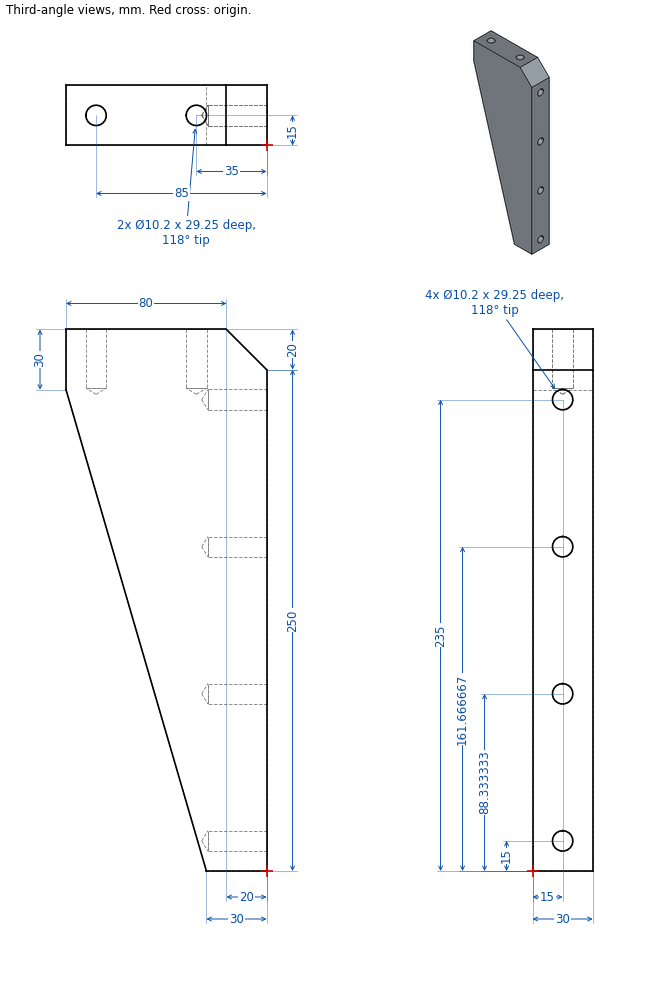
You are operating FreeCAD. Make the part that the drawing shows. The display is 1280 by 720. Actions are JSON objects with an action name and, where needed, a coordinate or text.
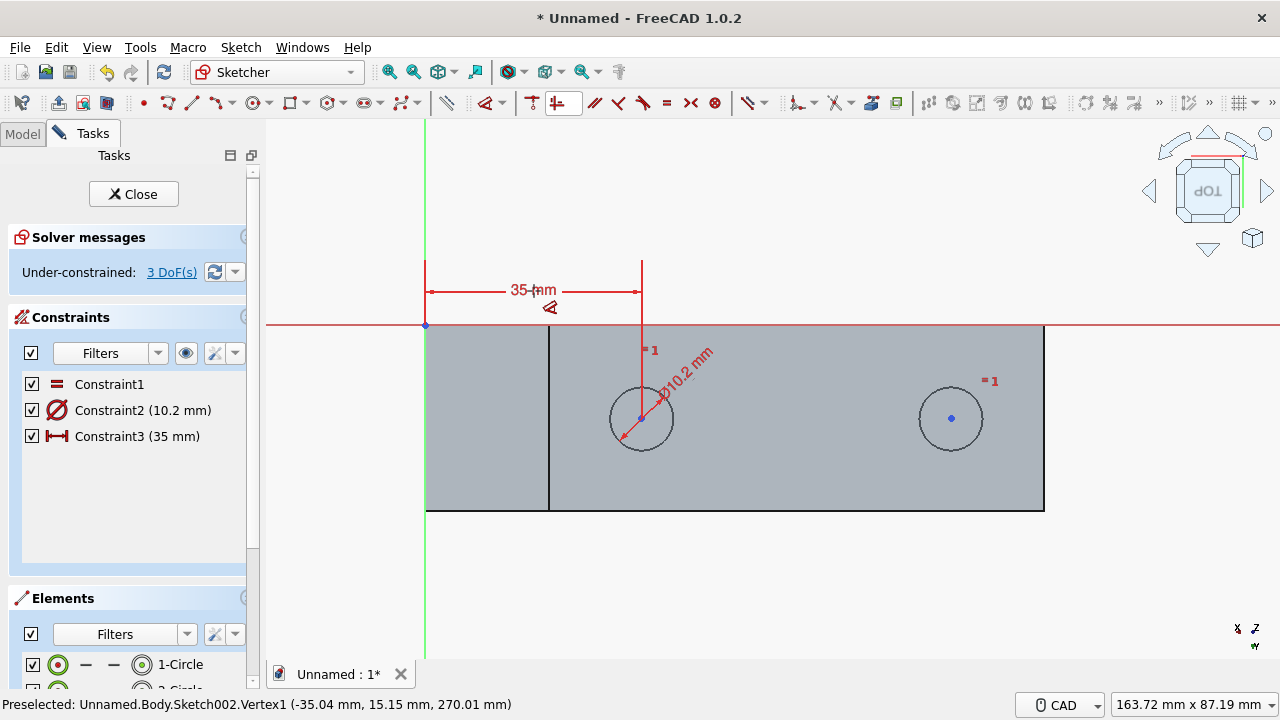
{"action": "left_click", "coordinate": [642, 419]}
{"action": "left_click", "coordinate": [391, 372]}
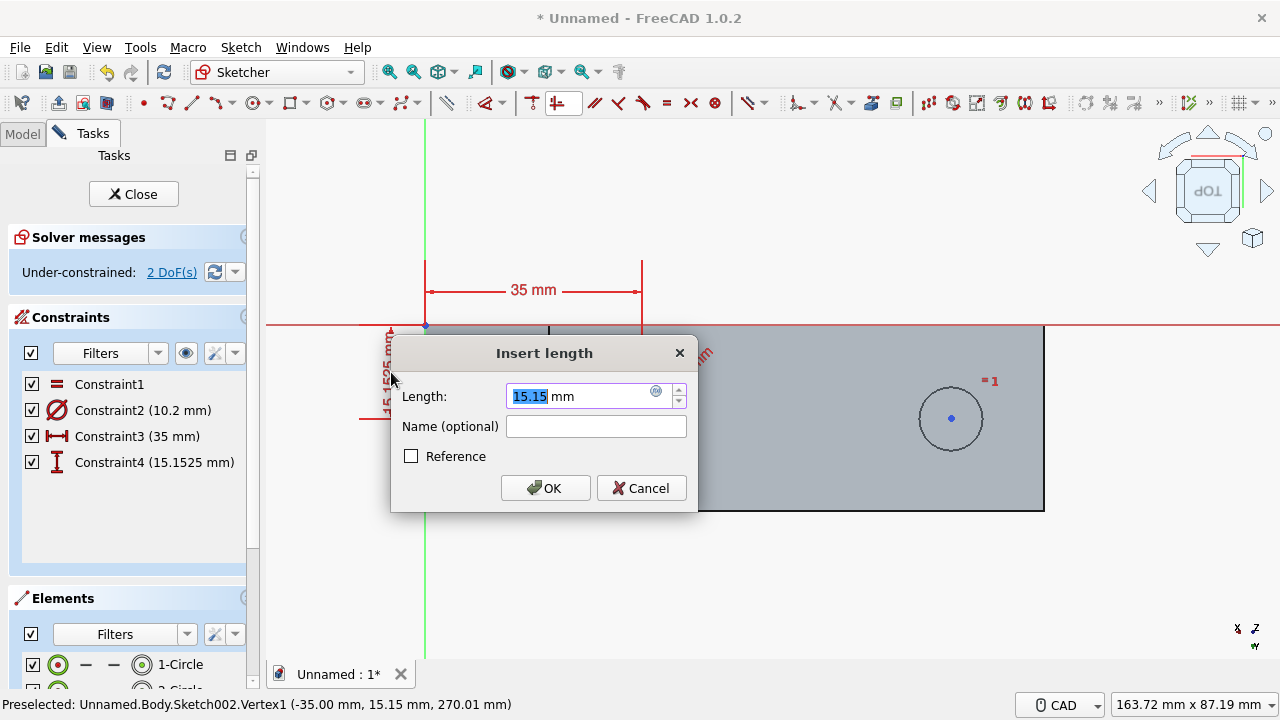
{"action": "type", "text": "15"}
{"action": "key", "text": "Return"}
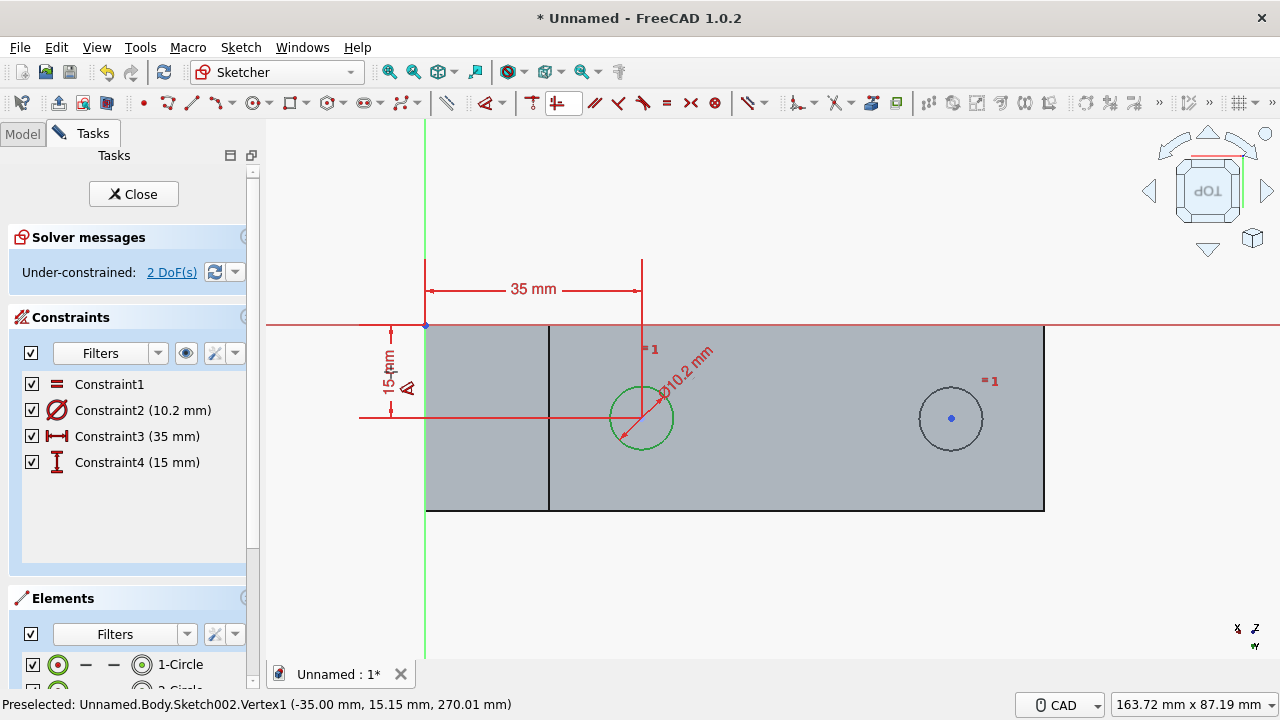
{"action": "left_click", "coordinate": [951, 419]}
{"action": "left_click", "coordinate": [688, 291]}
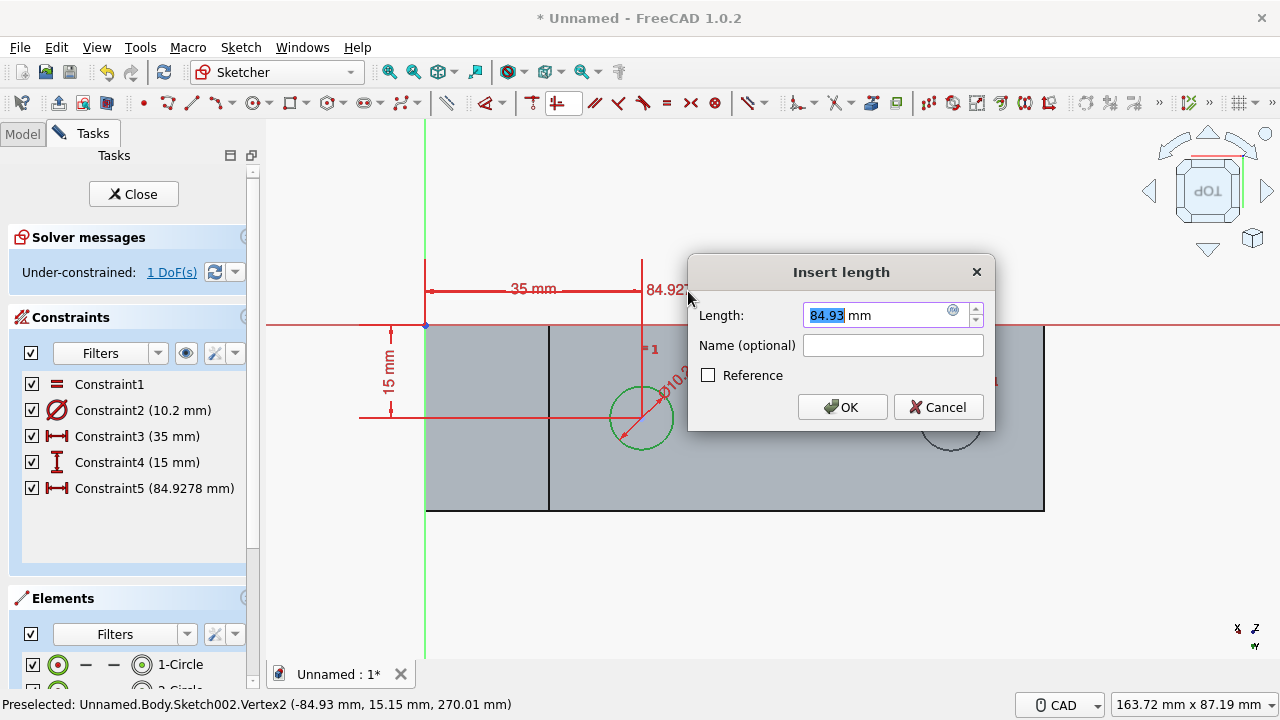
{"action": "type", "text": "85"}
{"action": "key", "text": "Return"}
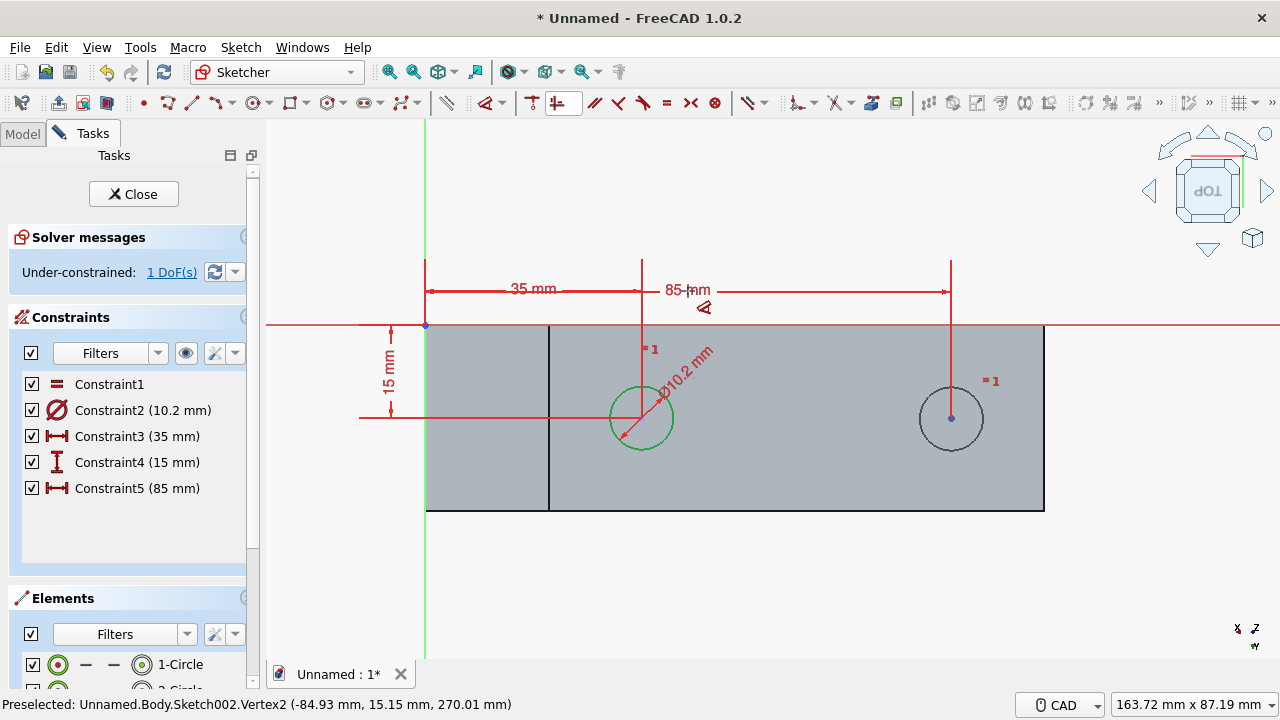
{"action": "left_click", "coordinate": [951, 419]}
{"action": "left_click", "coordinate": [391, 350]}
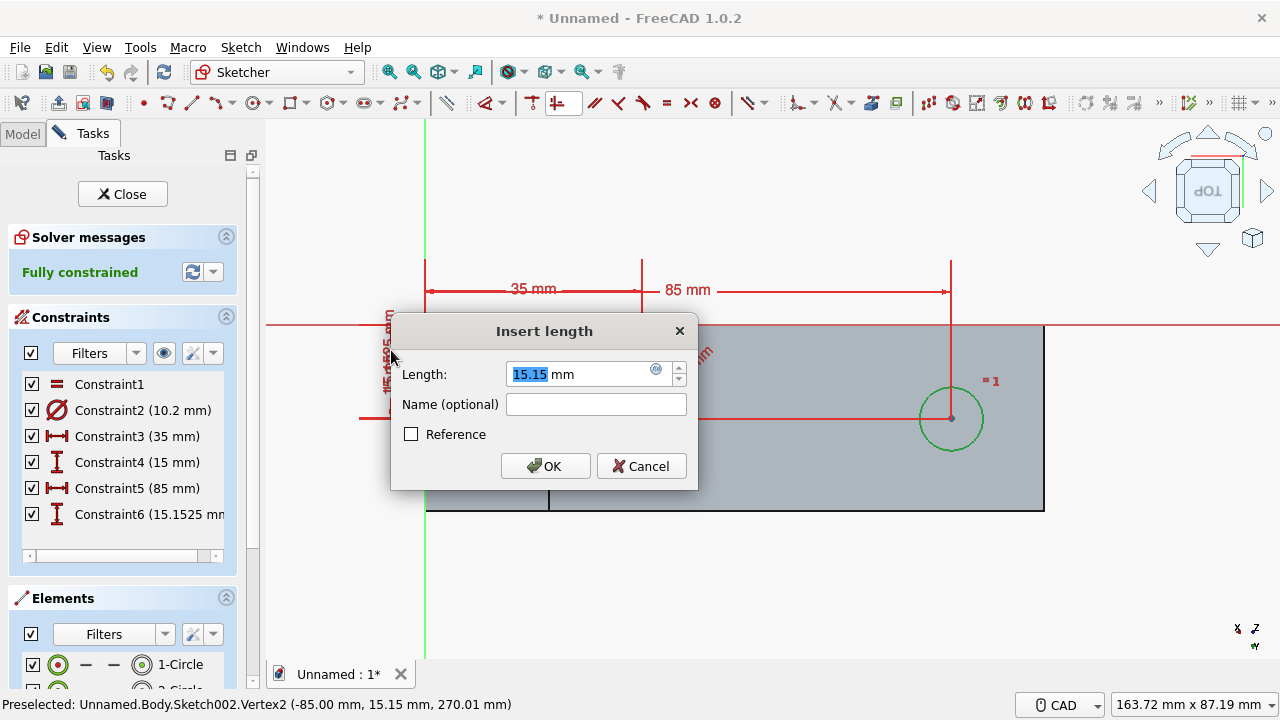
{"action": "type", "text": "15"}
{"action": "key", "text": "Return"}
{"action": "key", "text": "Escape"}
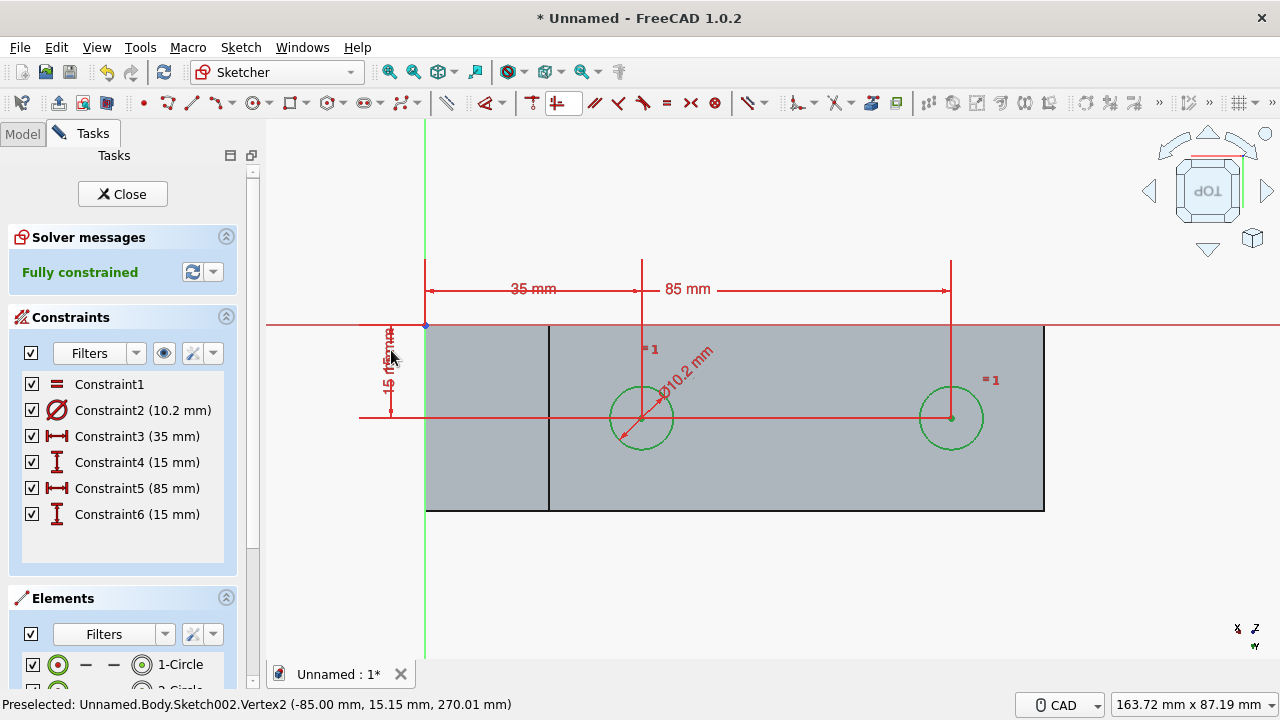
{"action": "left_click", "coordinate": [123, 194]}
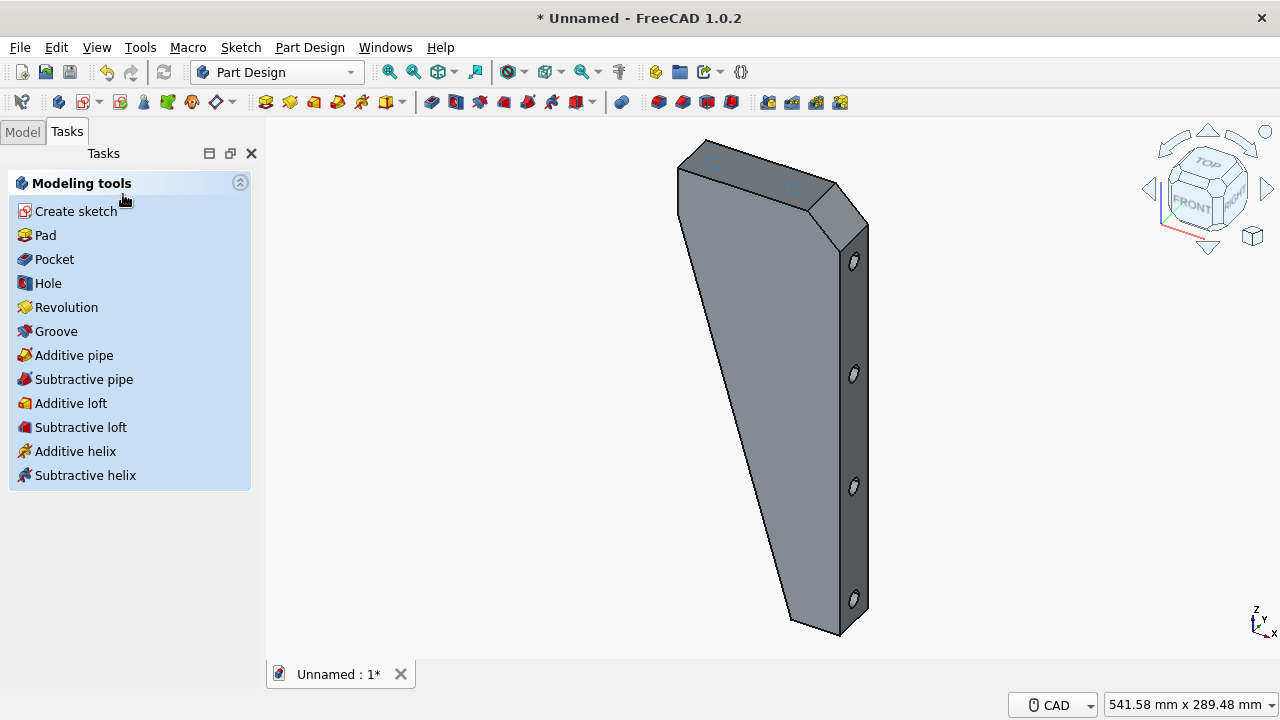
{"action": "left_click", "coordinate": [456, 102]}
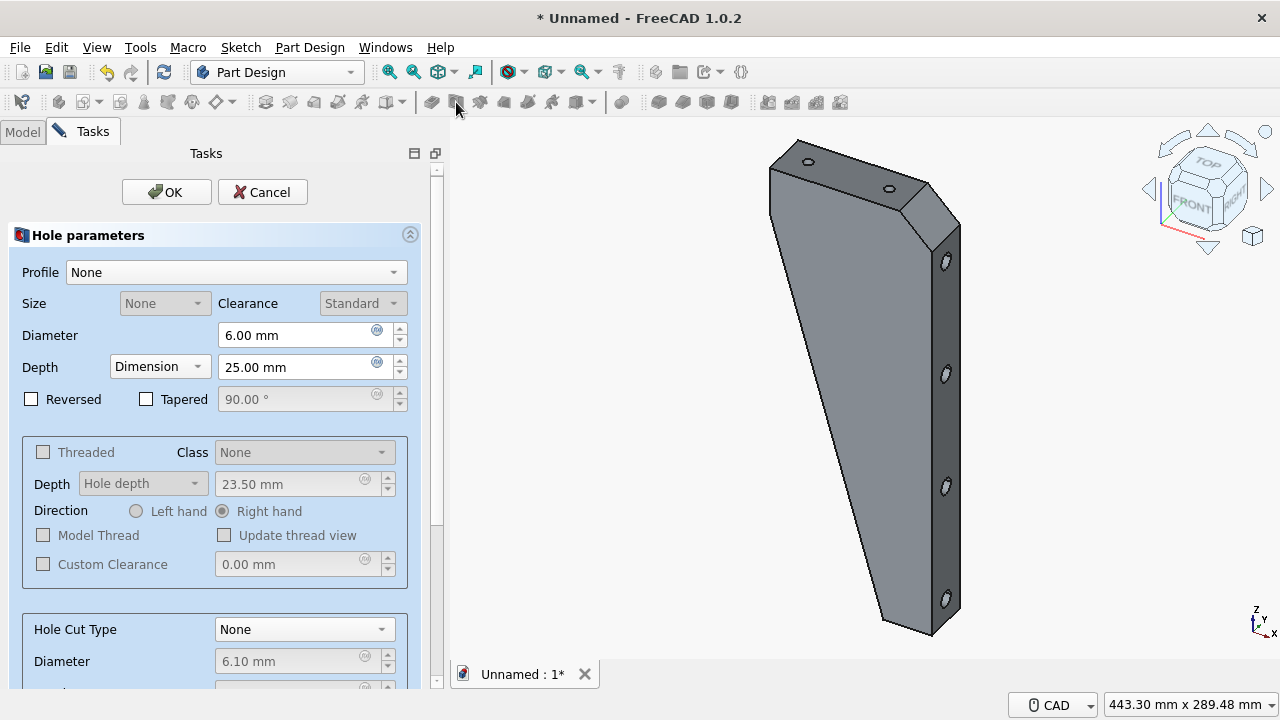
{"action": "triple_click", "coordinate": [305, 335]}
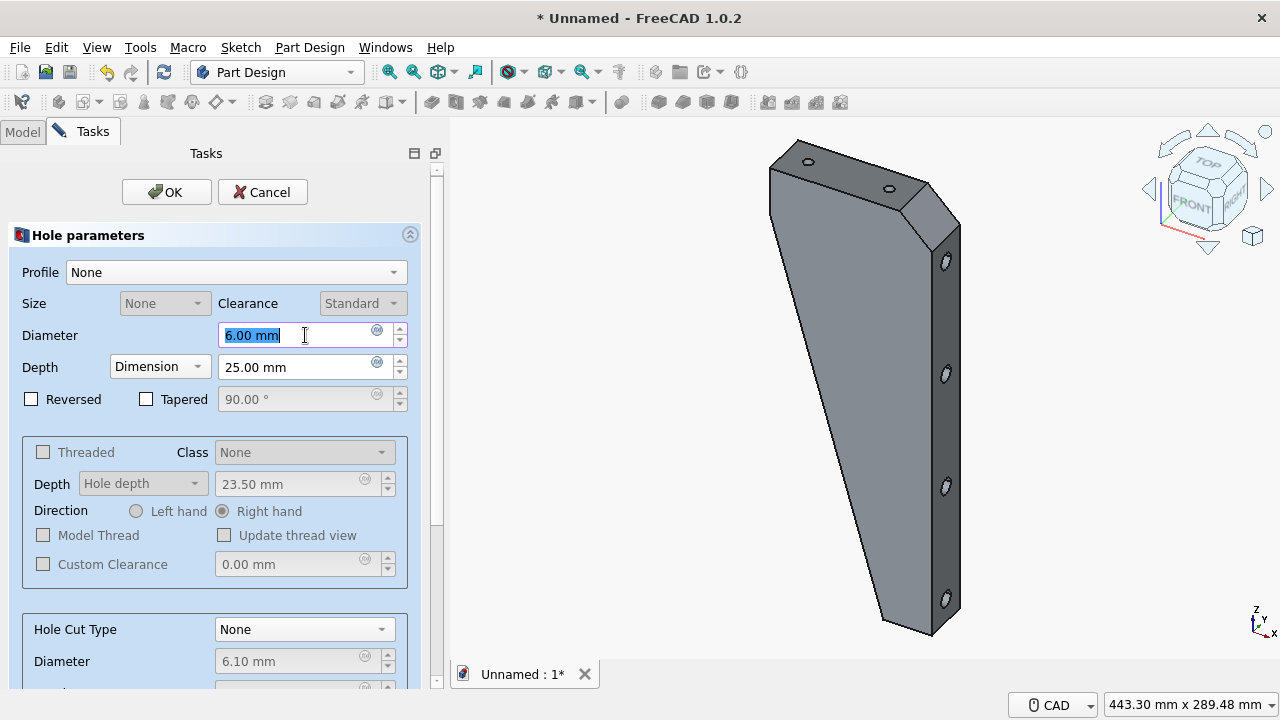
{"action": "type", "text": "10.2"}
{"action": "key", "text": "Tab"}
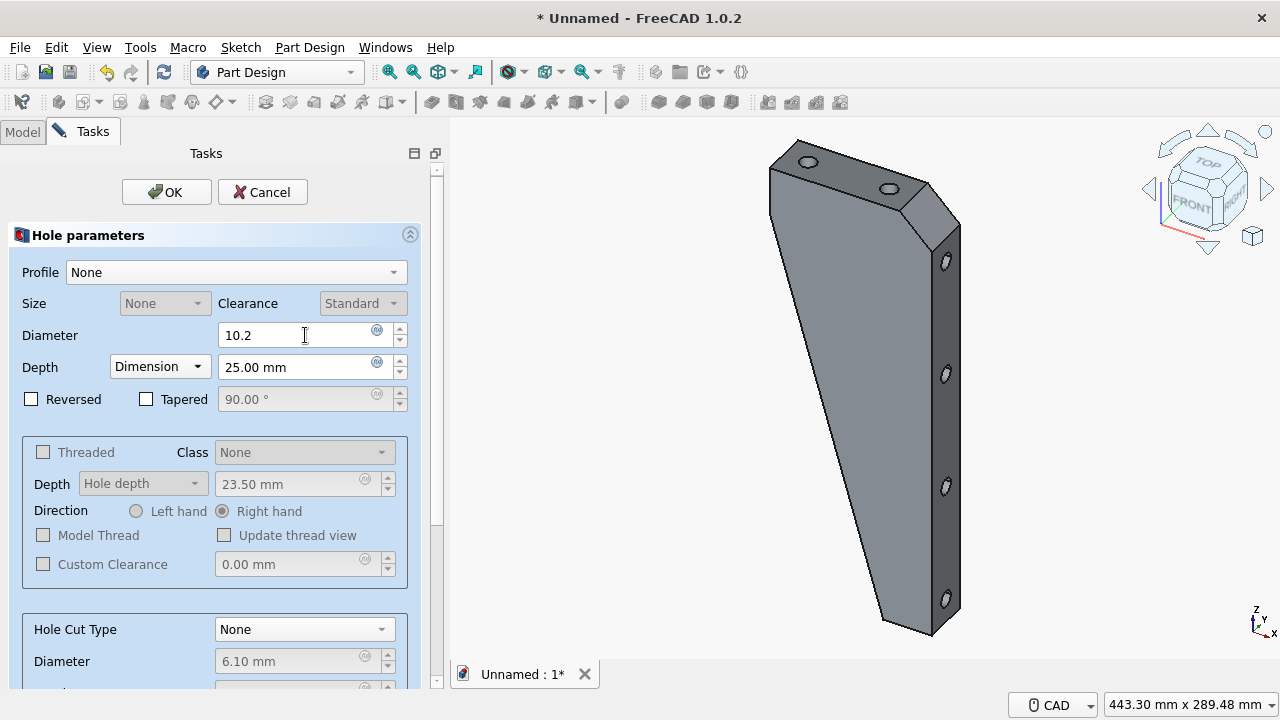
{"action": "triple_click", "coordinate": [305, 367]}